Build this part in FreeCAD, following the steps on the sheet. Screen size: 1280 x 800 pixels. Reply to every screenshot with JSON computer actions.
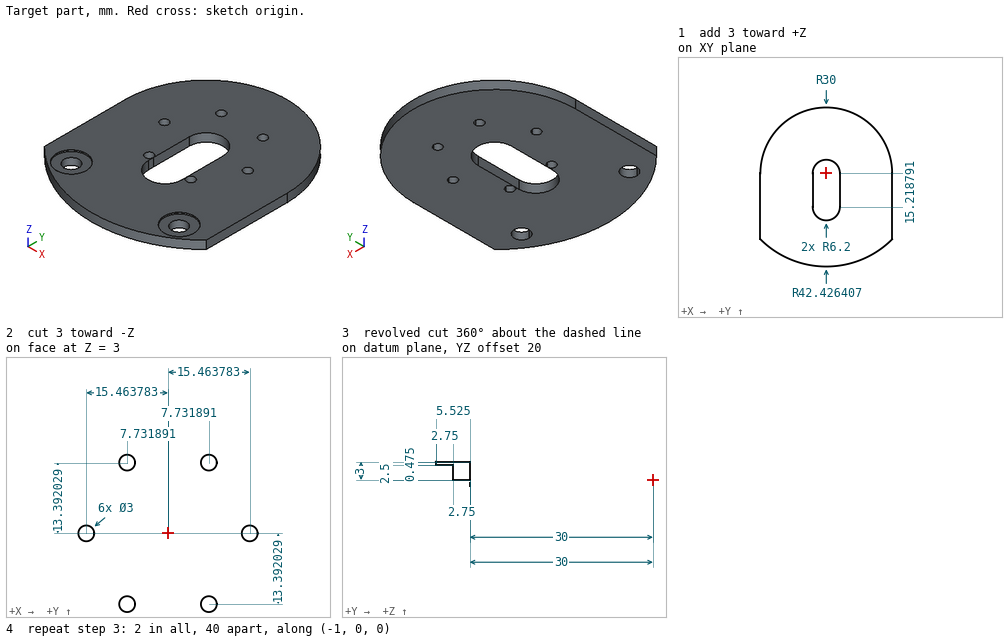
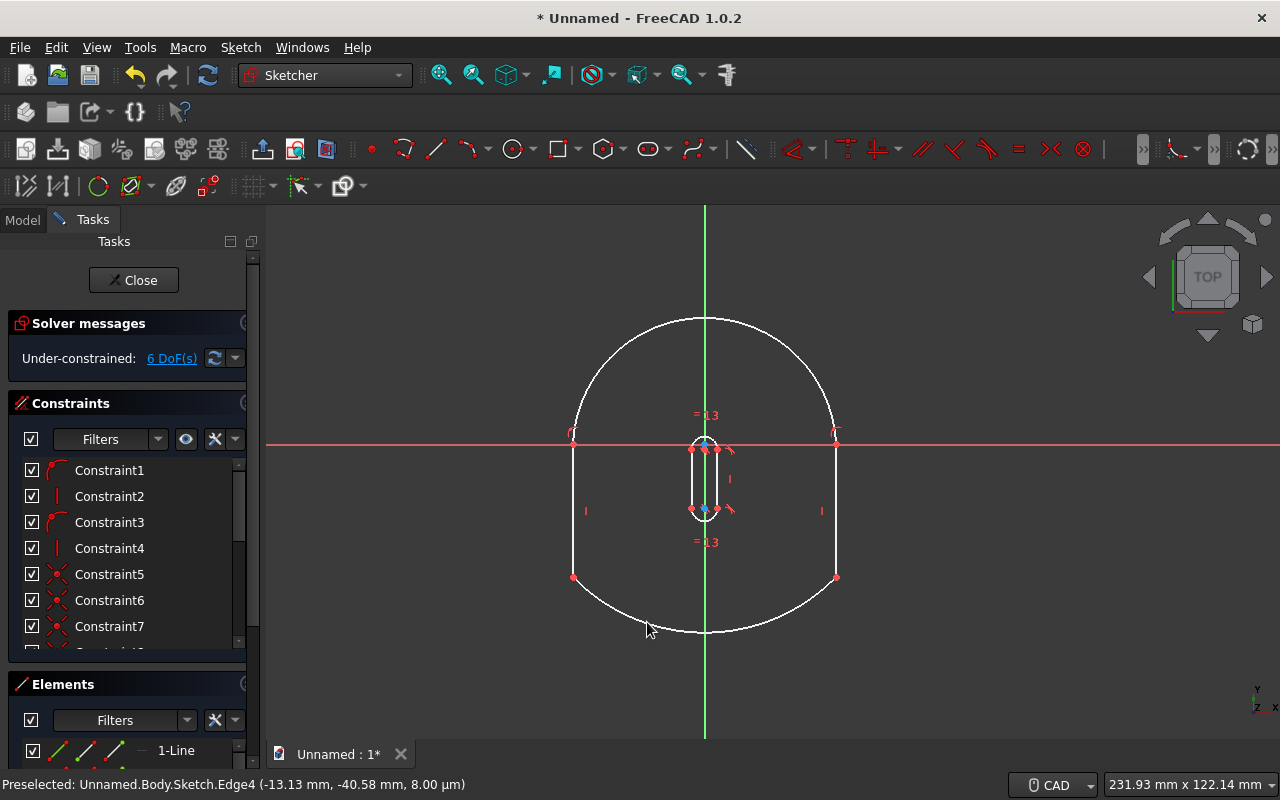
{"action": "scroll", "coordinate": [705, 447], "scroll_direction": "up", "scroll_amount": 6}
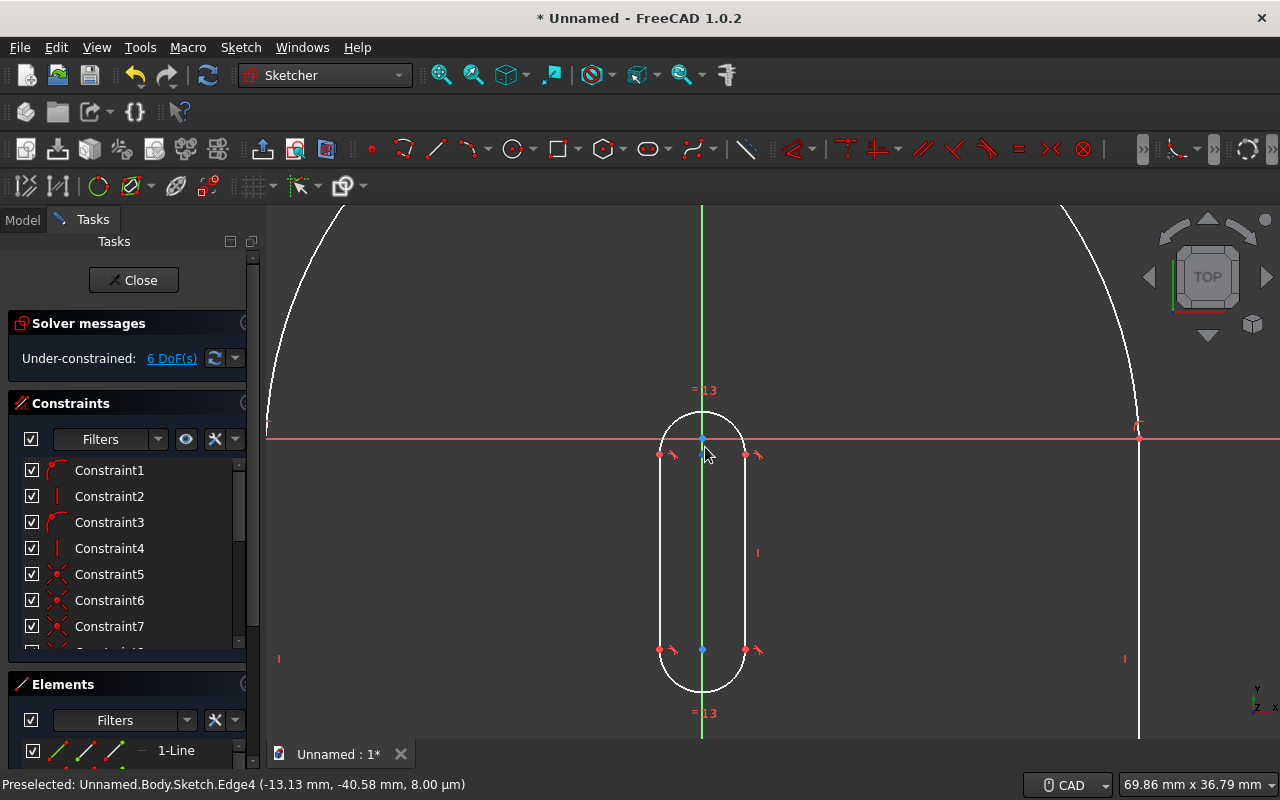
{"action": "left_click_drag", "start_coordinate": [692, 429], "coordinate": [712, 464]}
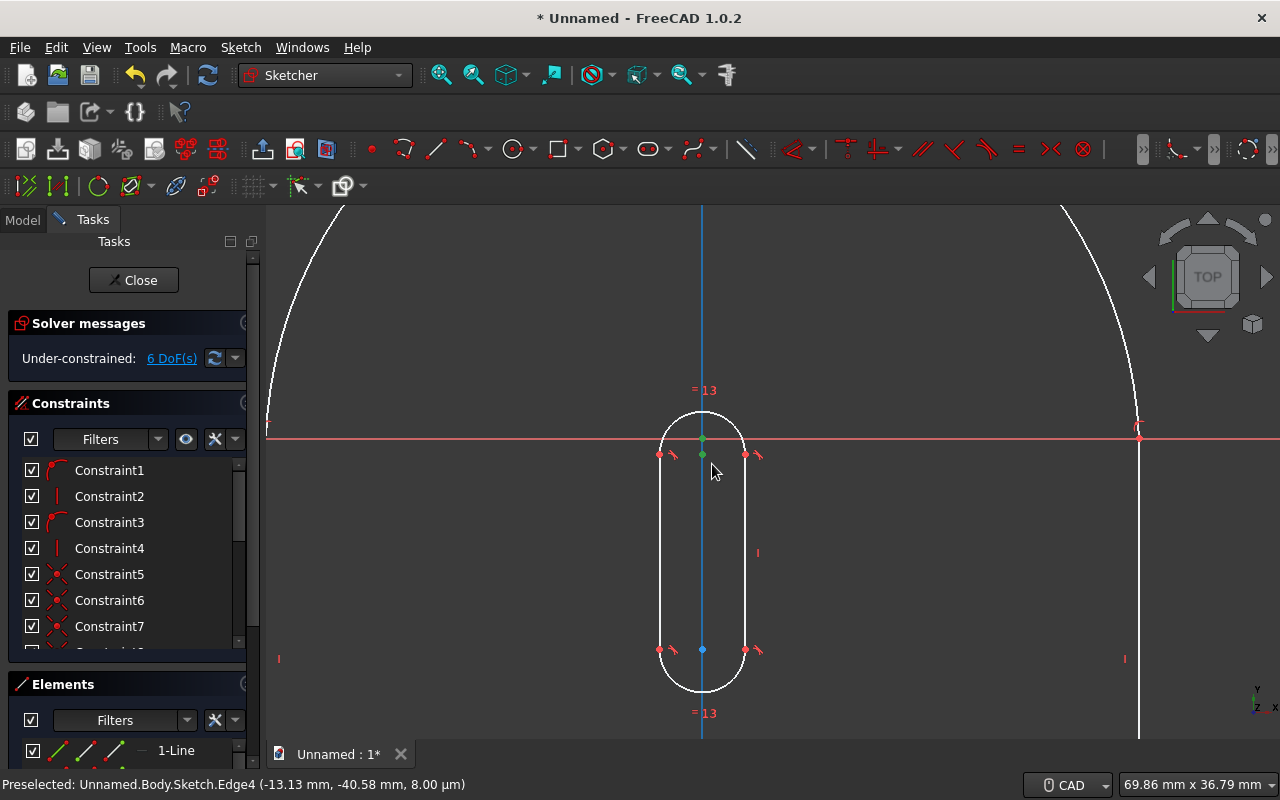
{"action": "key", "text": "c"}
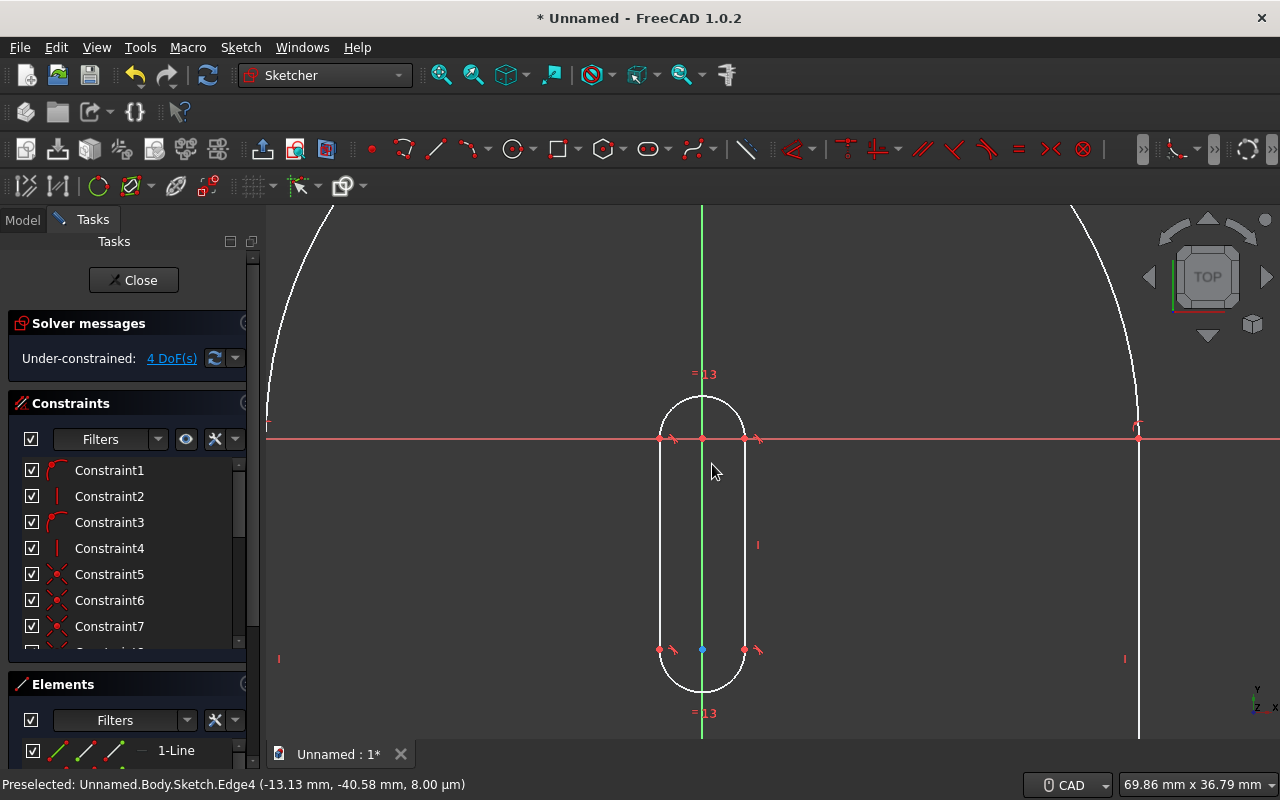
{"action": "key", "text": "d"}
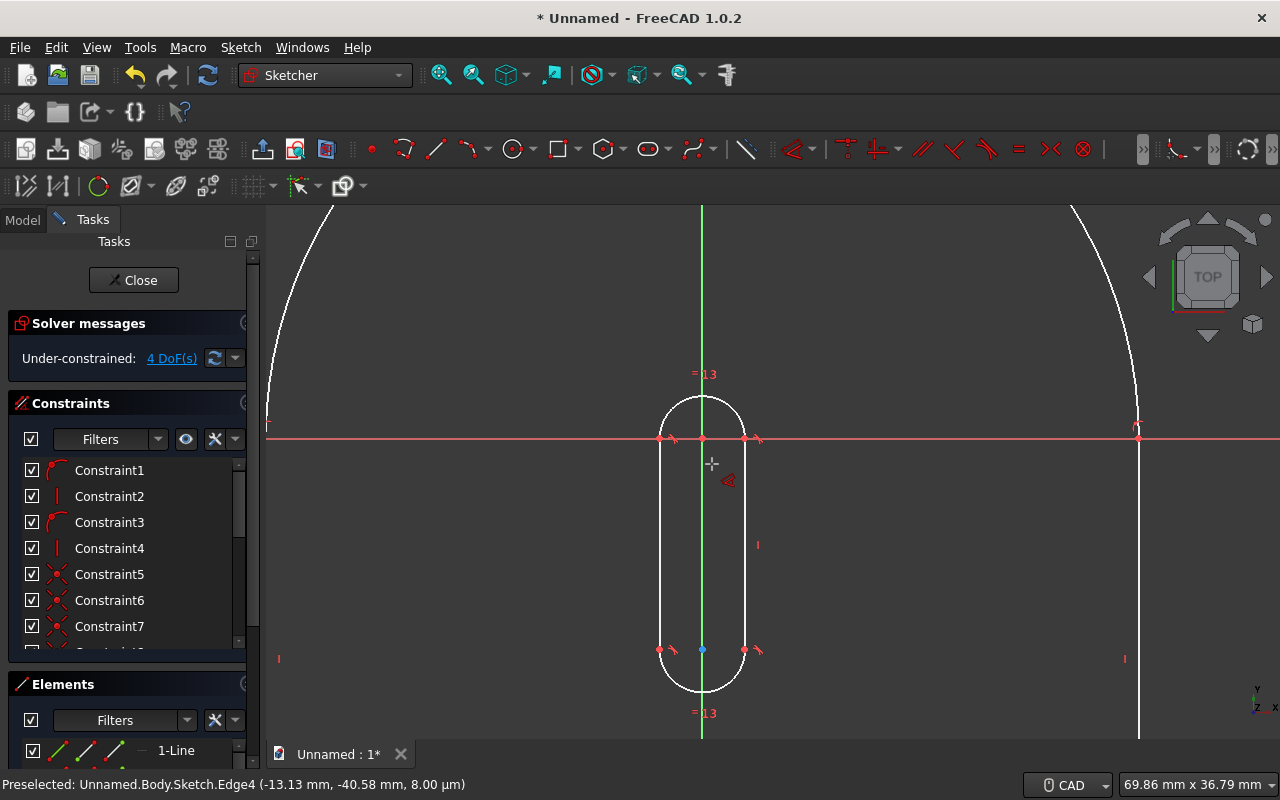
{"action": "scroll", "coordinate": [705, 447], "scroll_direction": "down", "scroll_amount": 6}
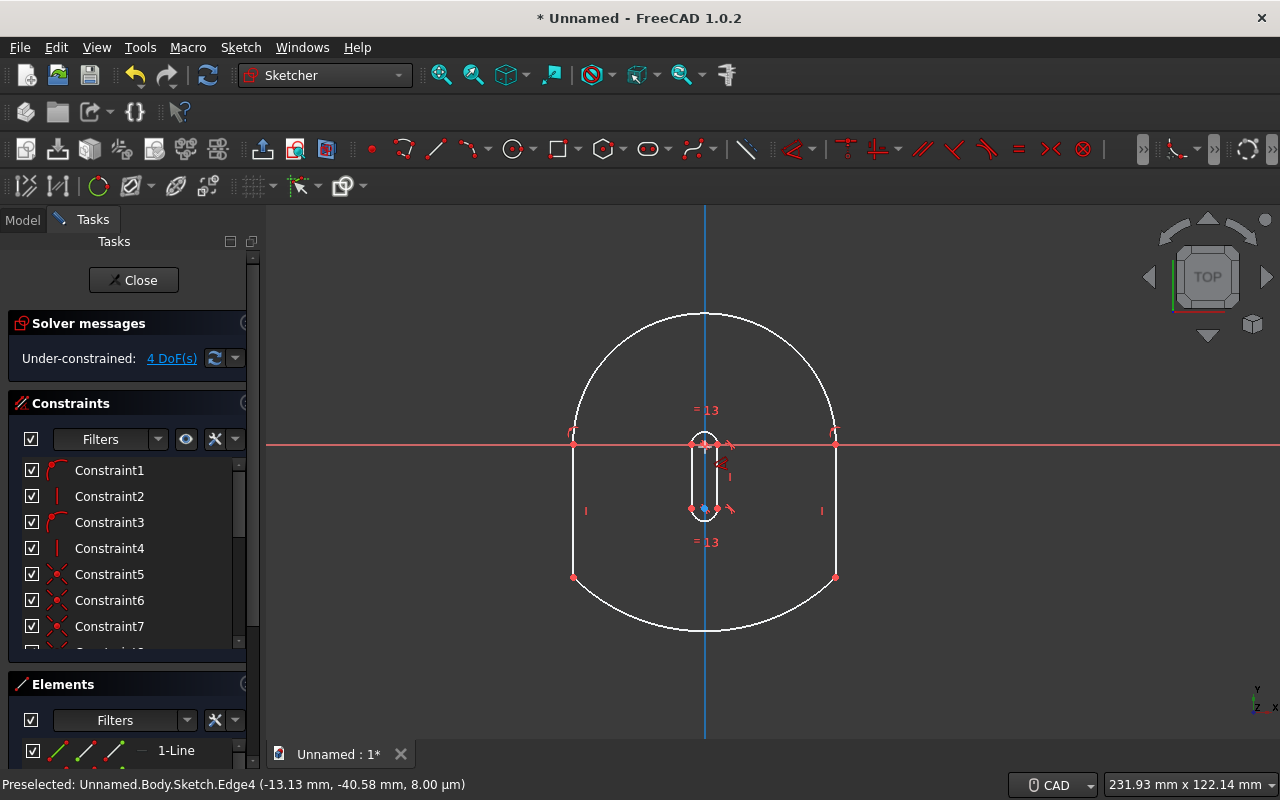
{"action": "left_click", "coordinate": [782, 338]}
{"action": "left_click", "coordinate": [801, 312]}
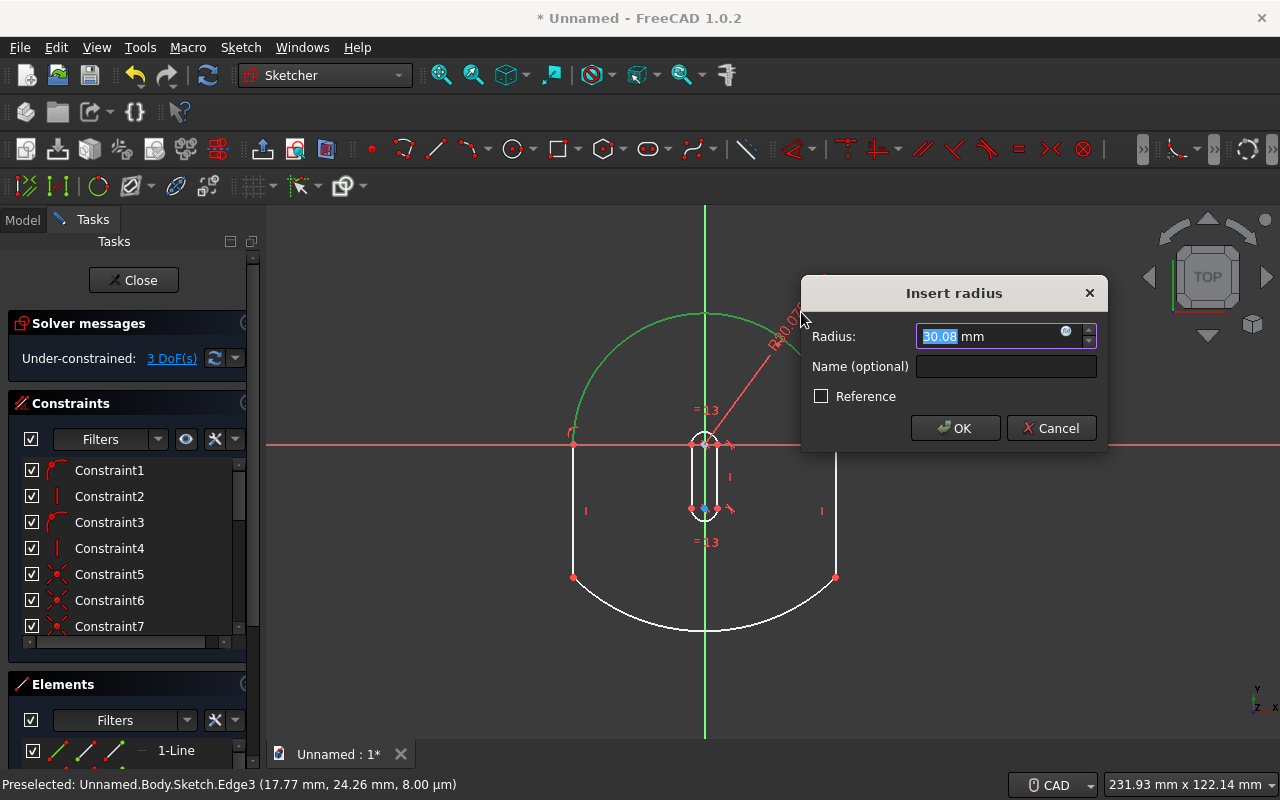
{"action": "type", "text": "30"}
{"action": "key", "text": "Return"}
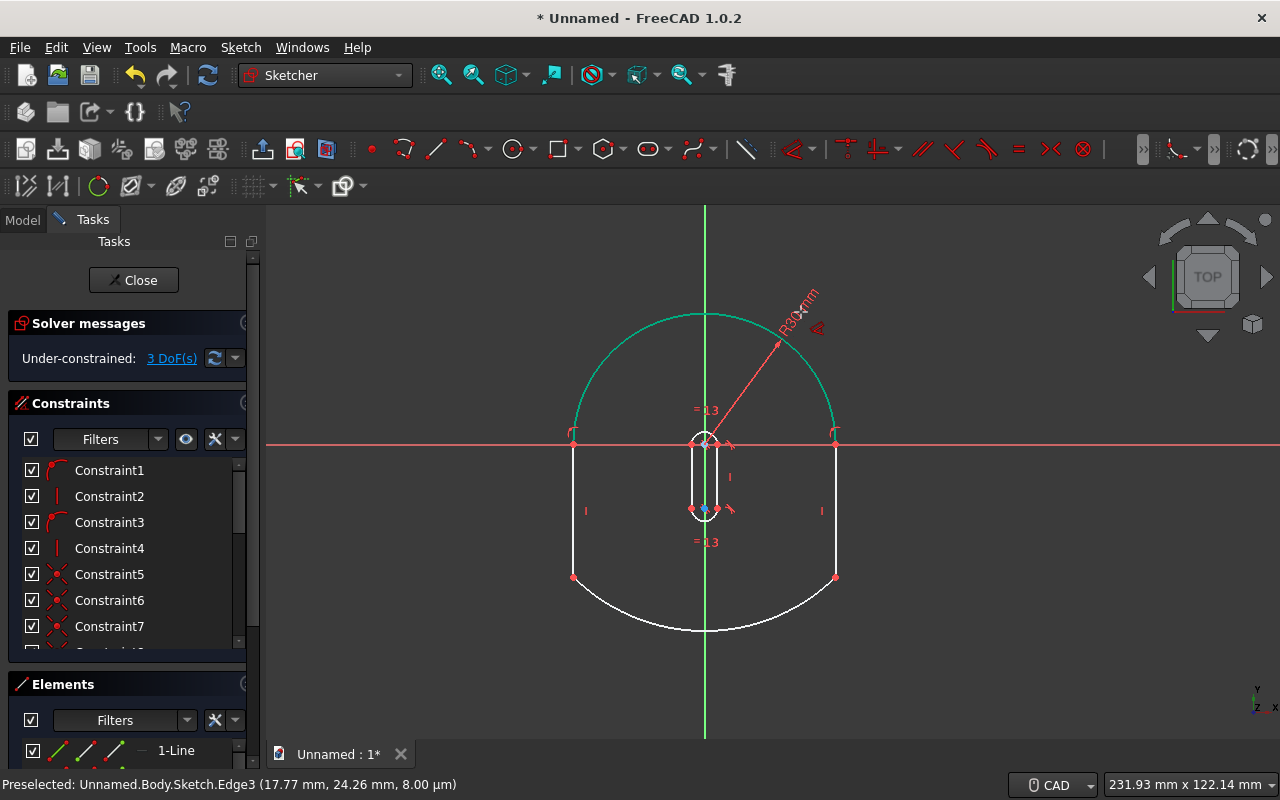
{"action": "left_click", "coordinate": [647, 622]}
{"action": "left_click", "coordinate": [637, 652]}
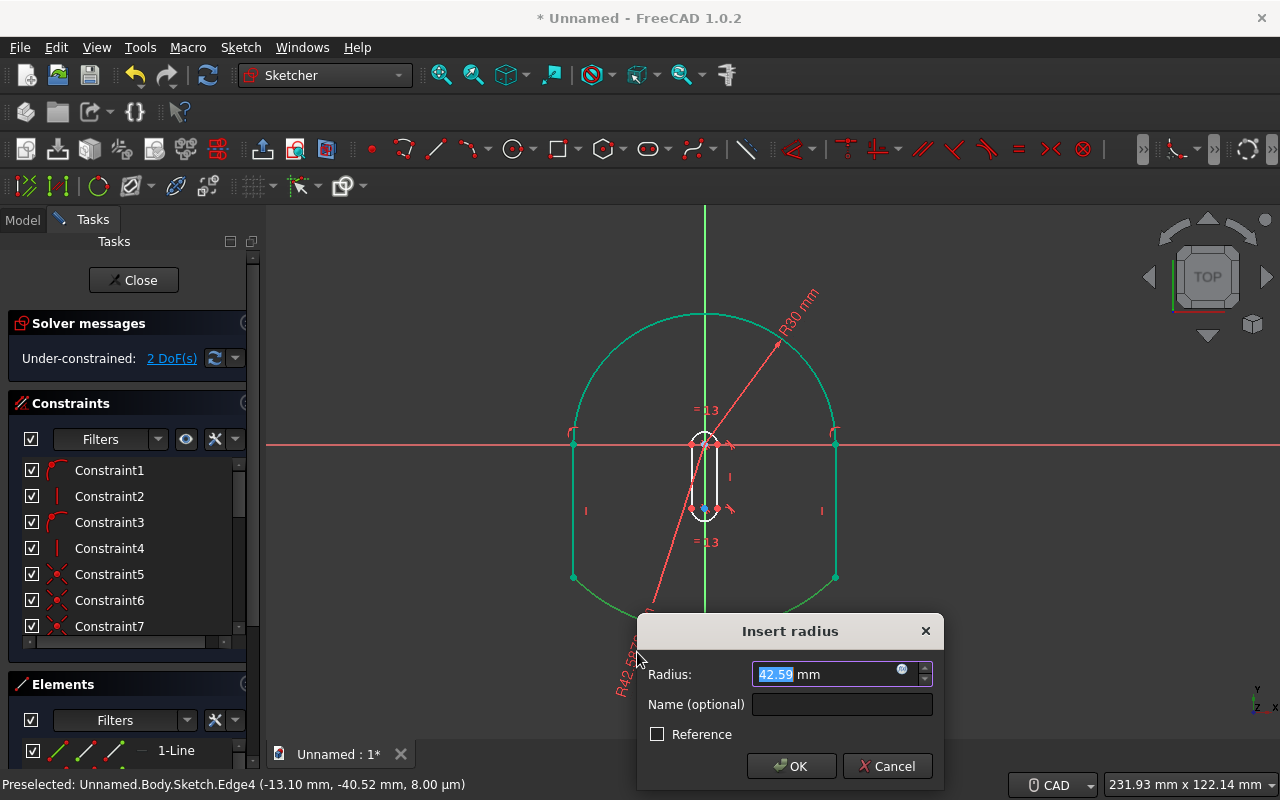
{"action": "type", "text": "42.426407"}
{"action": "key", "text": "Return"}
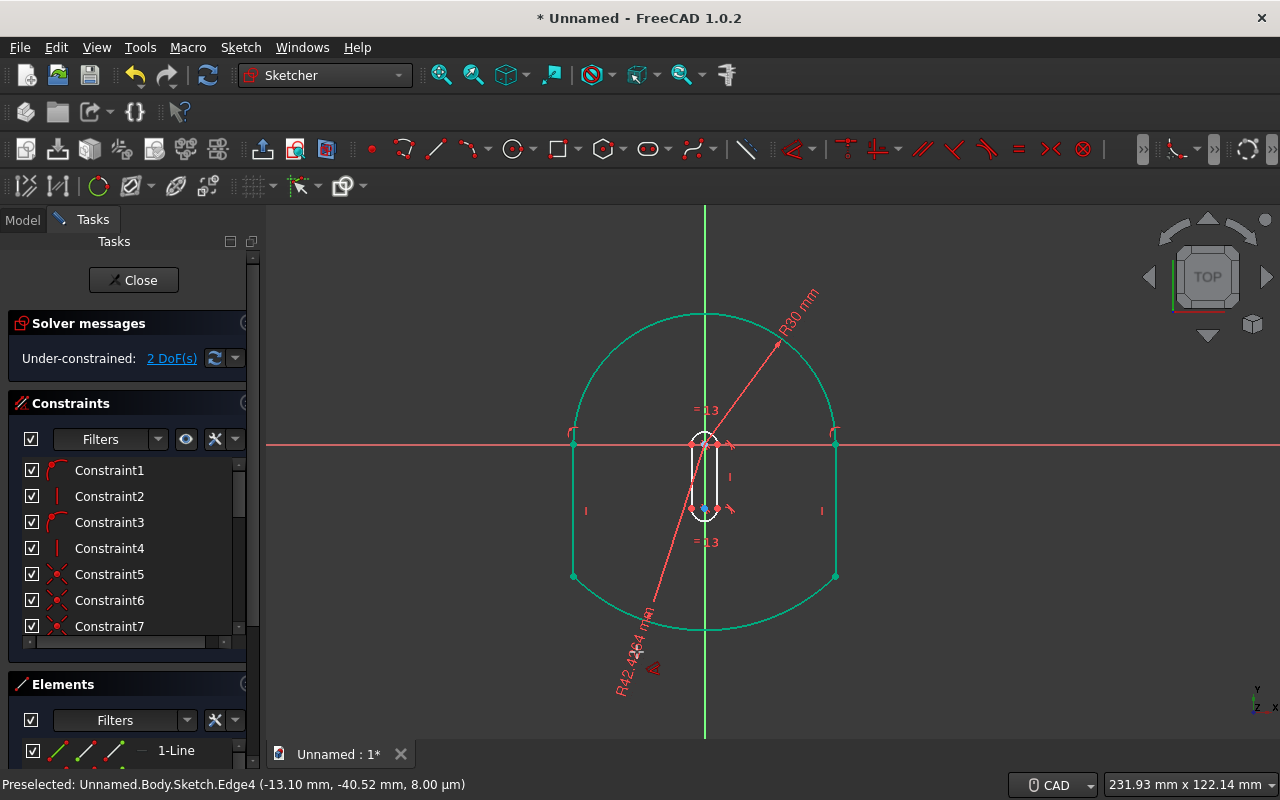
{"action": "scroll", "coordinate": [705, 432], "scroll_direction": "up", "scroll_amount": 2}